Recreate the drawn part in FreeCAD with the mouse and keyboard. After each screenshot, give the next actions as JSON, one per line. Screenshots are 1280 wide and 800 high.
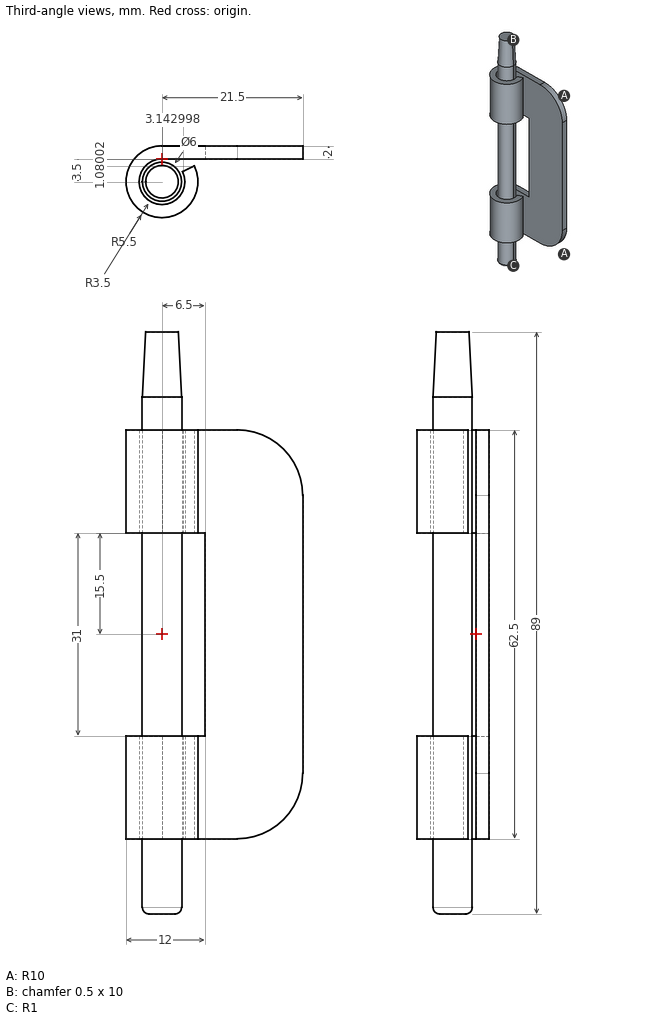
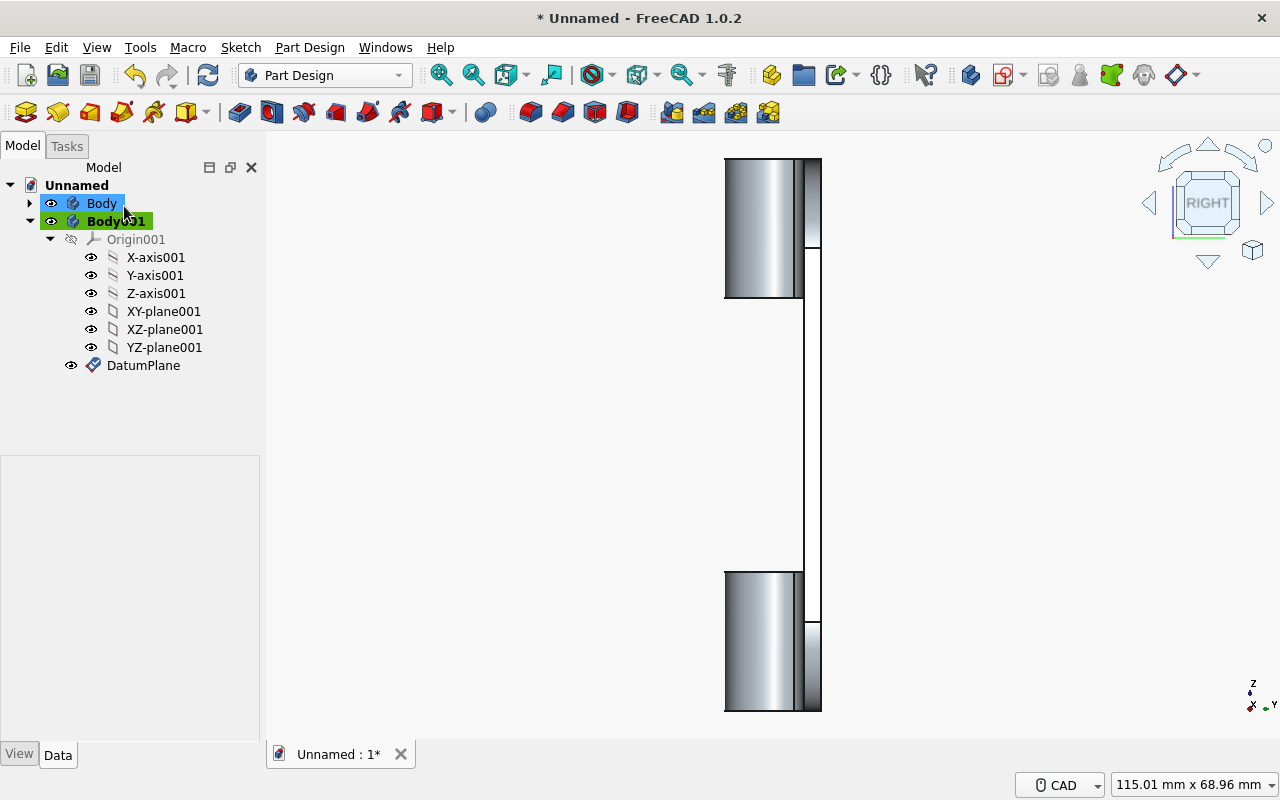
{"action": "left_click", "coordinate": [116, 365]}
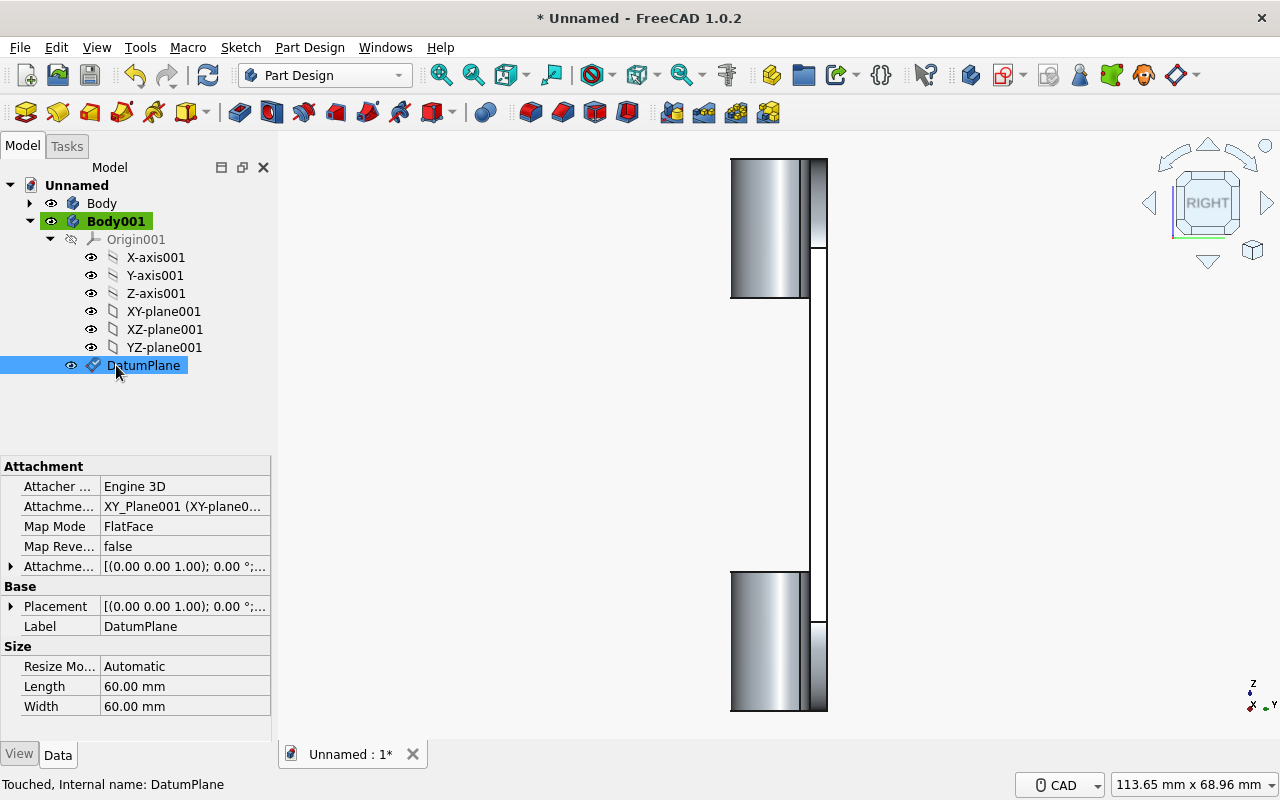
{"action": "left_click", "coordinate": [1004, 76]}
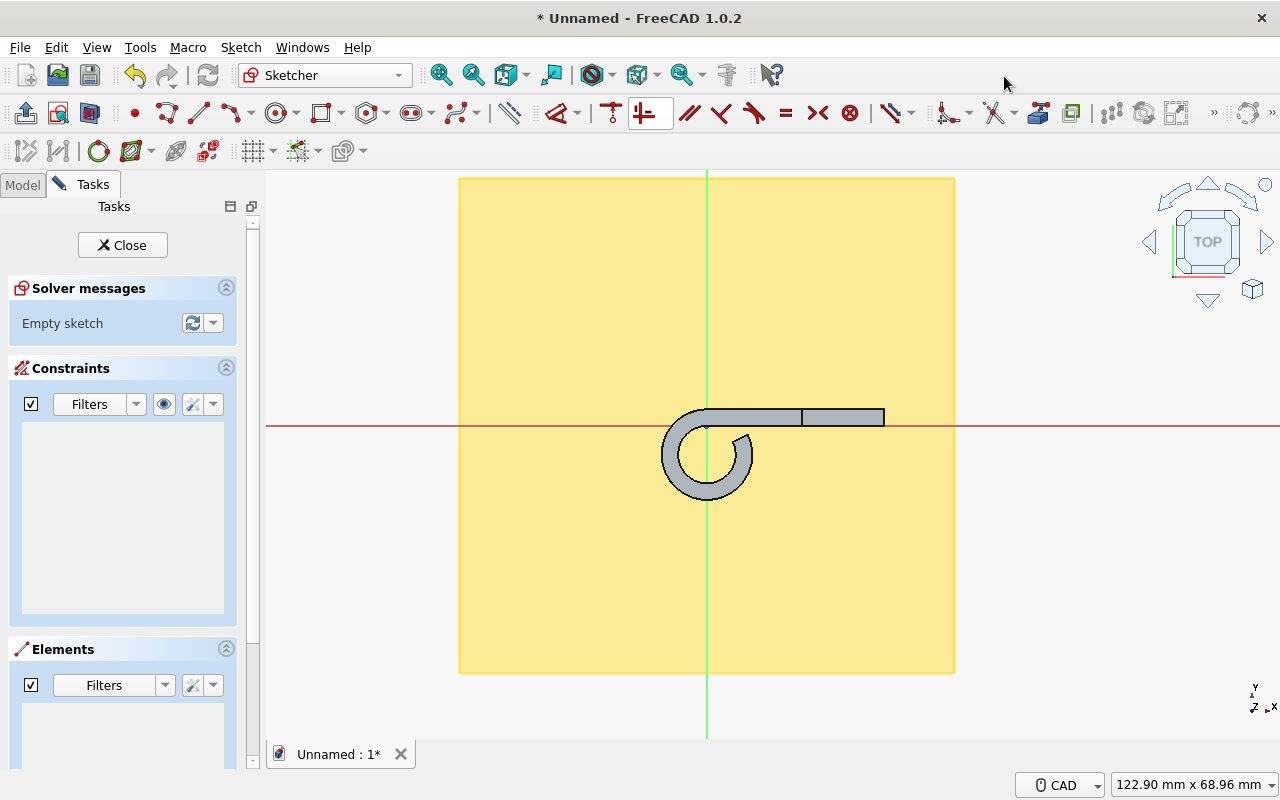
{"action": "scroll", "coordinate": [707, 452], "scroll_direction": "up", "scroll_amount": 10}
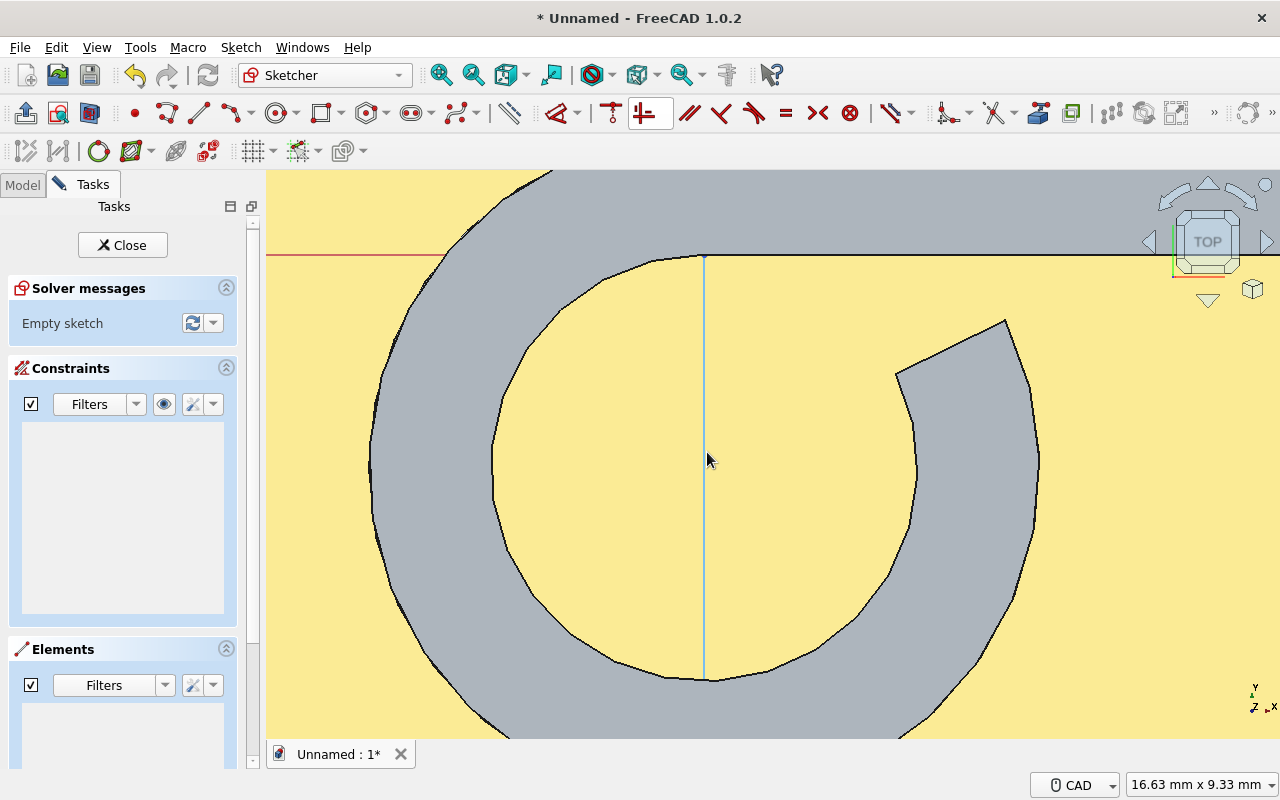
{"action": "left_click", "coordinate": [276, 114]}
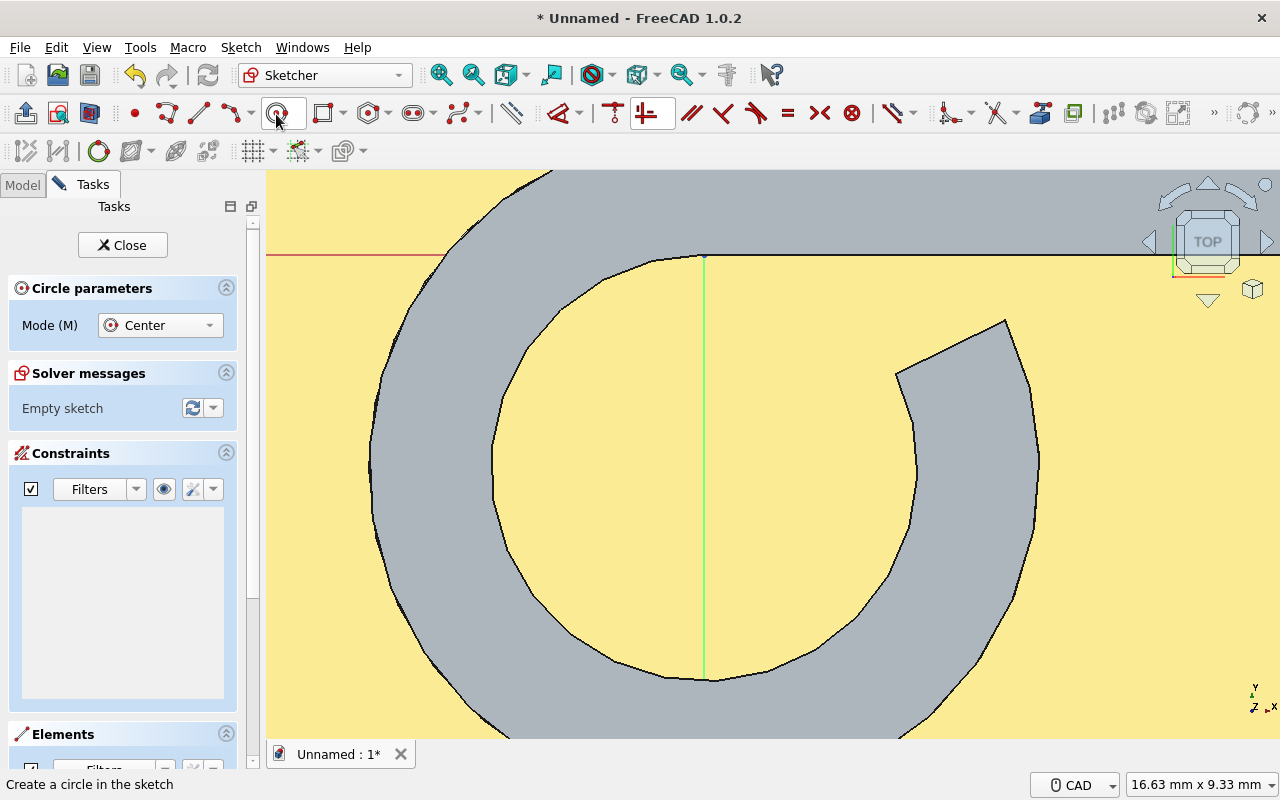
{"action": "left_click", "coordinate": [704, 468]}
{"action": "mouse_move", "coordinate": [833, 339]}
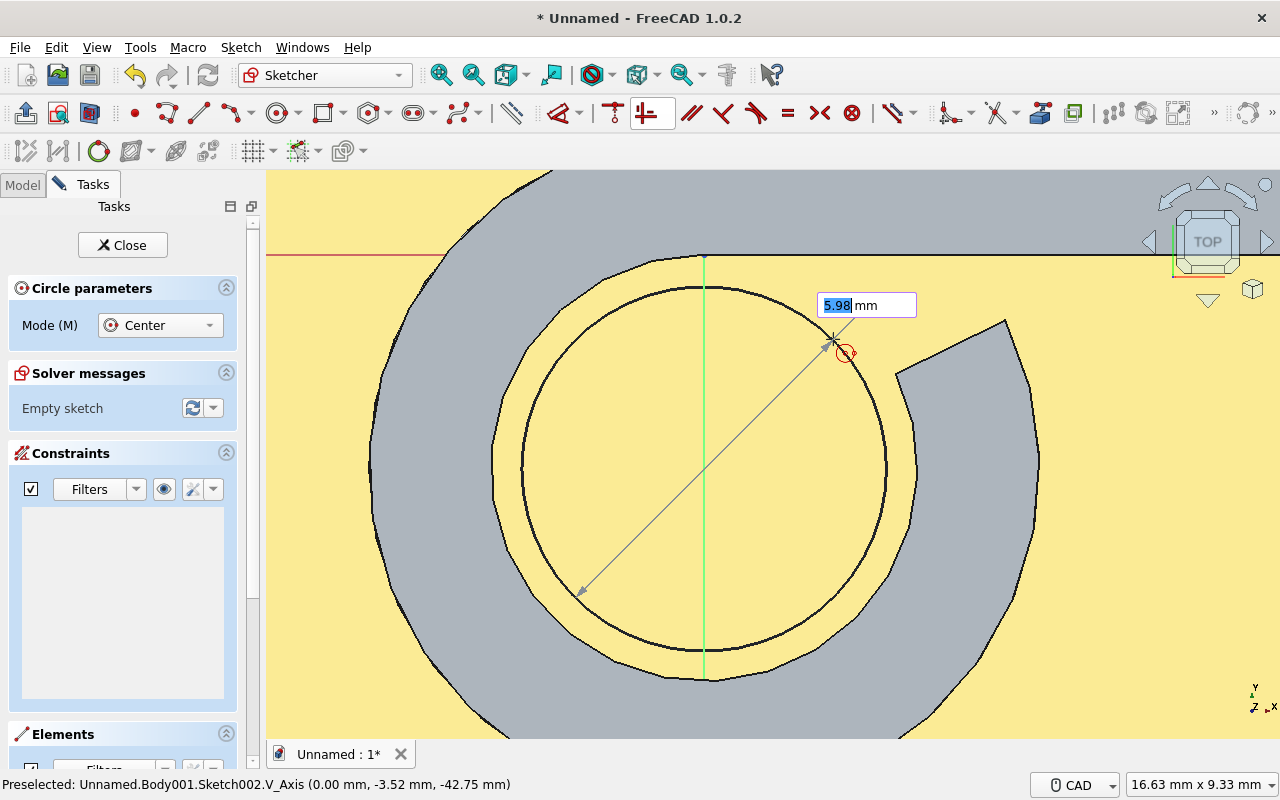
{"action": "type", "text": "6"}
{"action": "key", "text": "Return"}
{"action": "key", "text": "Escape"}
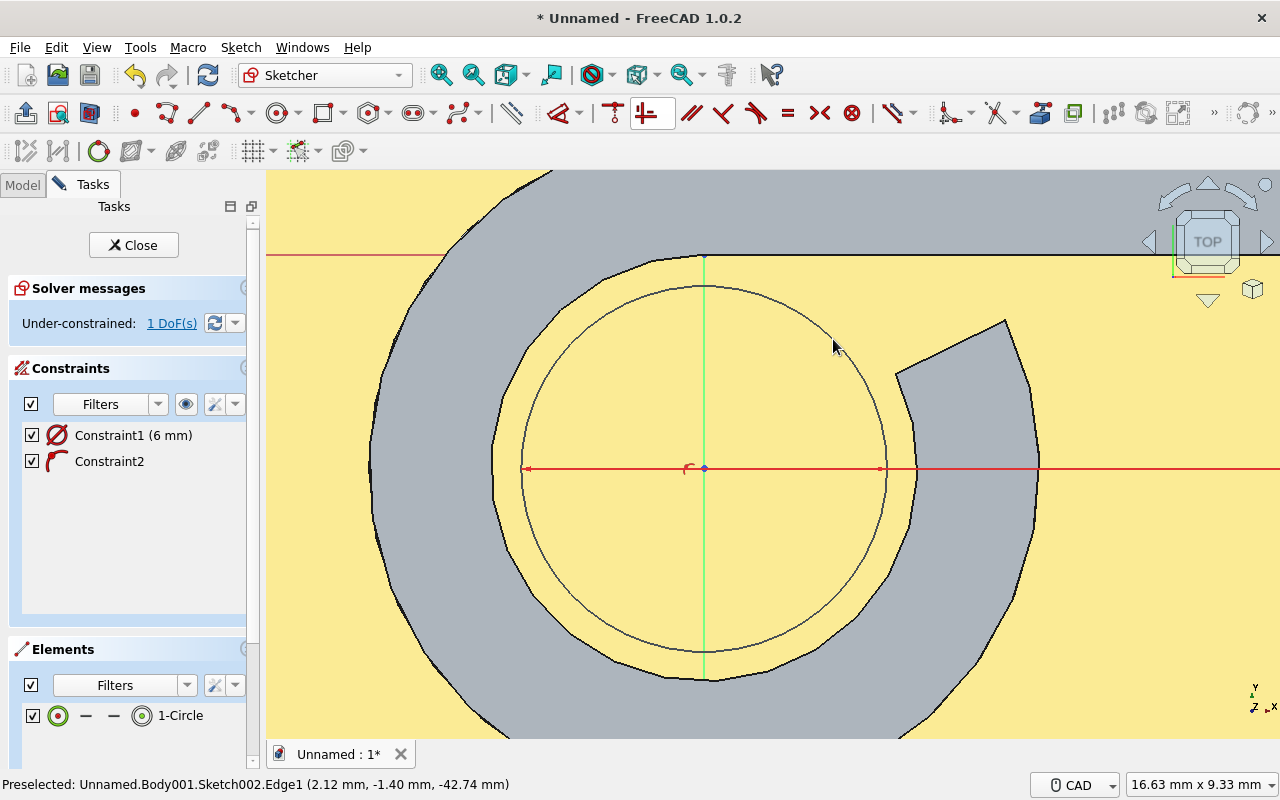
{"action": "key", "text": "d"}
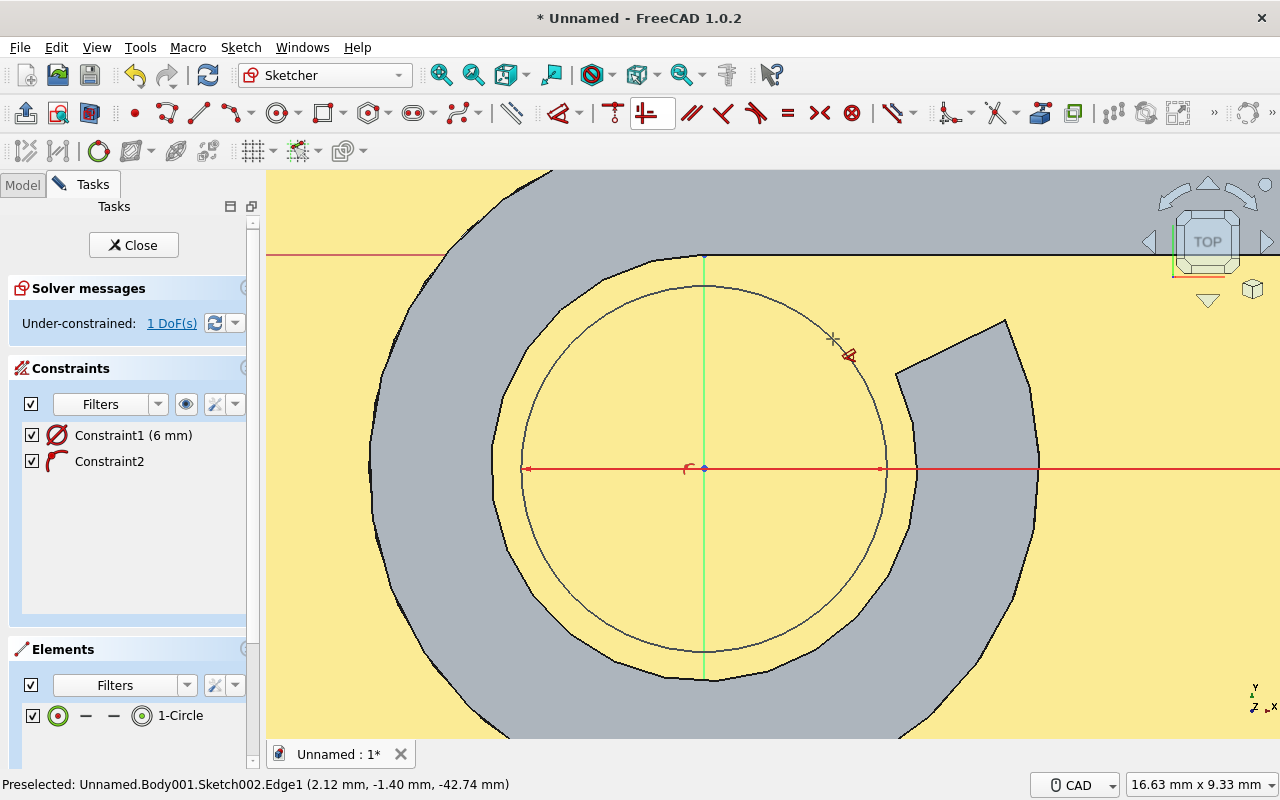
{"action": "left_click", "coordinate": [704, 469]}
{"action": "left_click", "coordinate": [738, 362]}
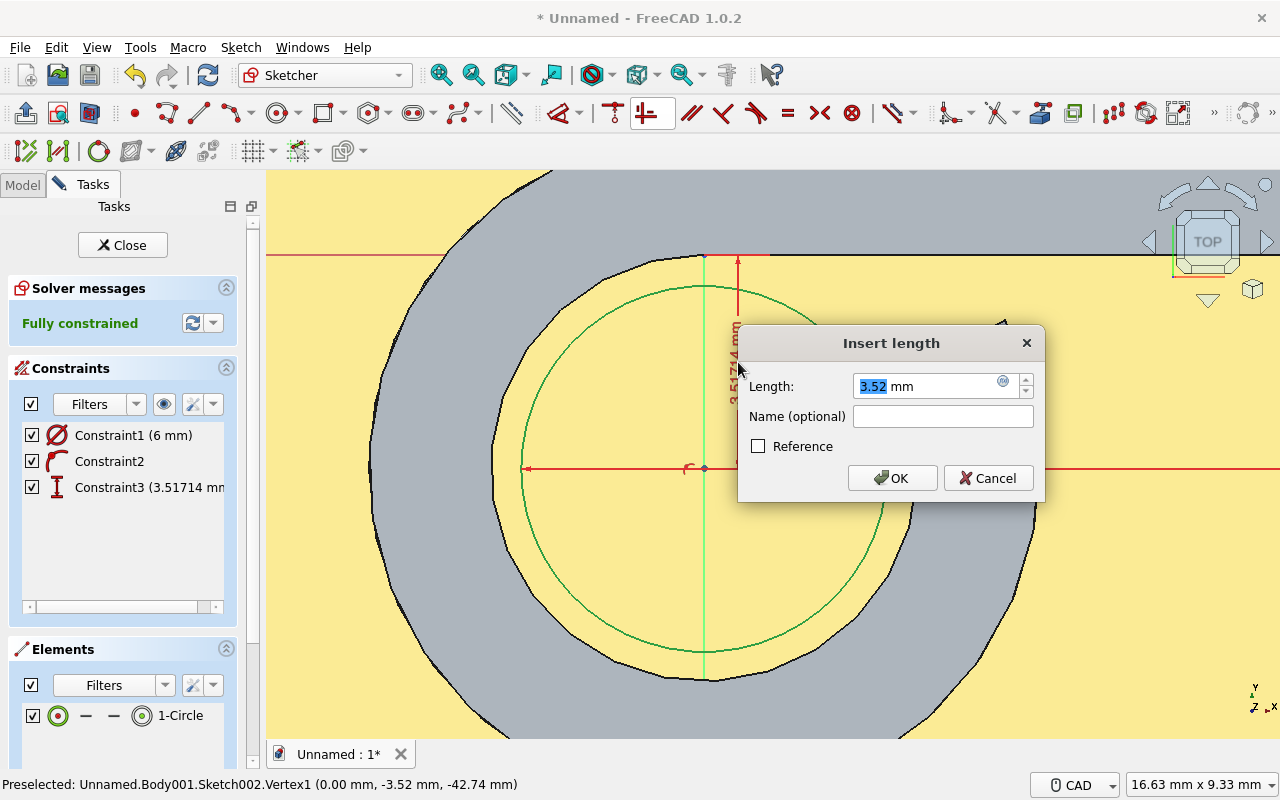
{"action": "type", "text": "3.5"}
{"action": "key", "text": "Return"}
{"action": "key", "text": "Escape"}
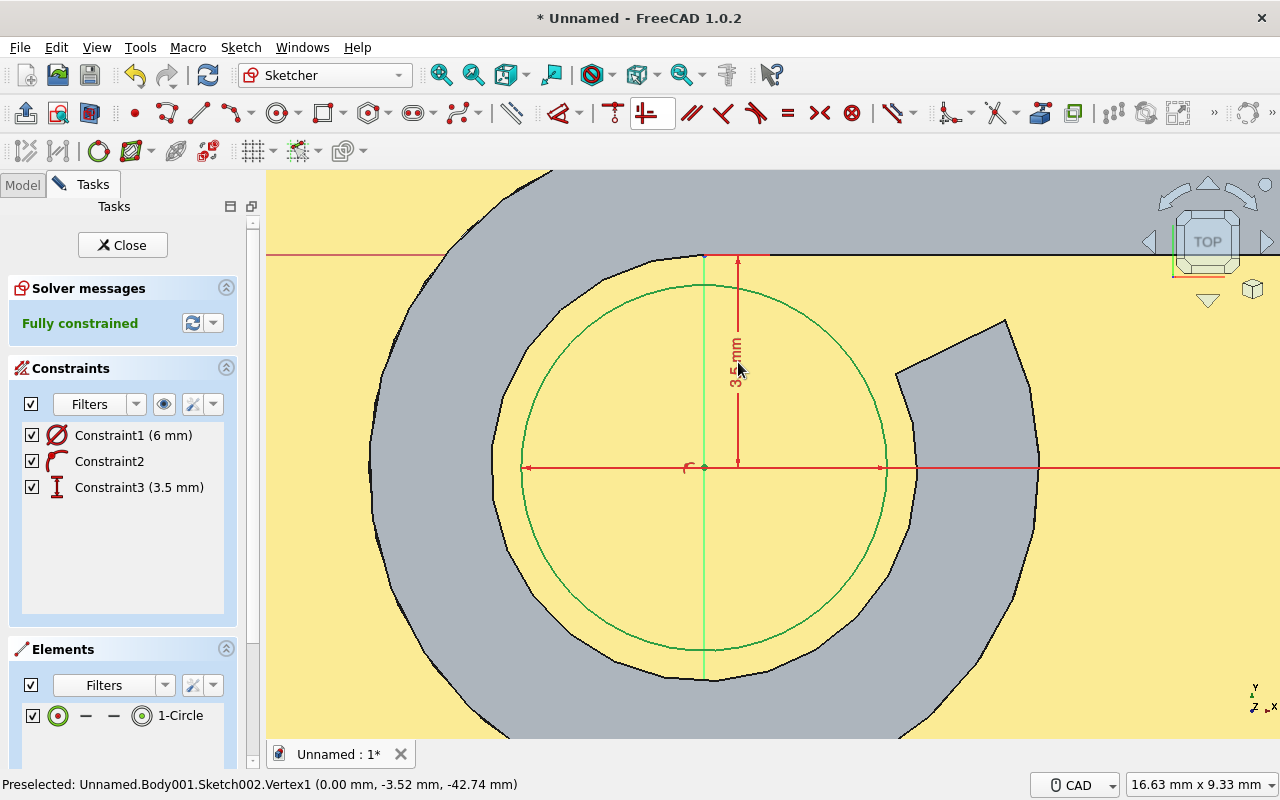
{"action": "left_click", "coordinate": [123, 245]}